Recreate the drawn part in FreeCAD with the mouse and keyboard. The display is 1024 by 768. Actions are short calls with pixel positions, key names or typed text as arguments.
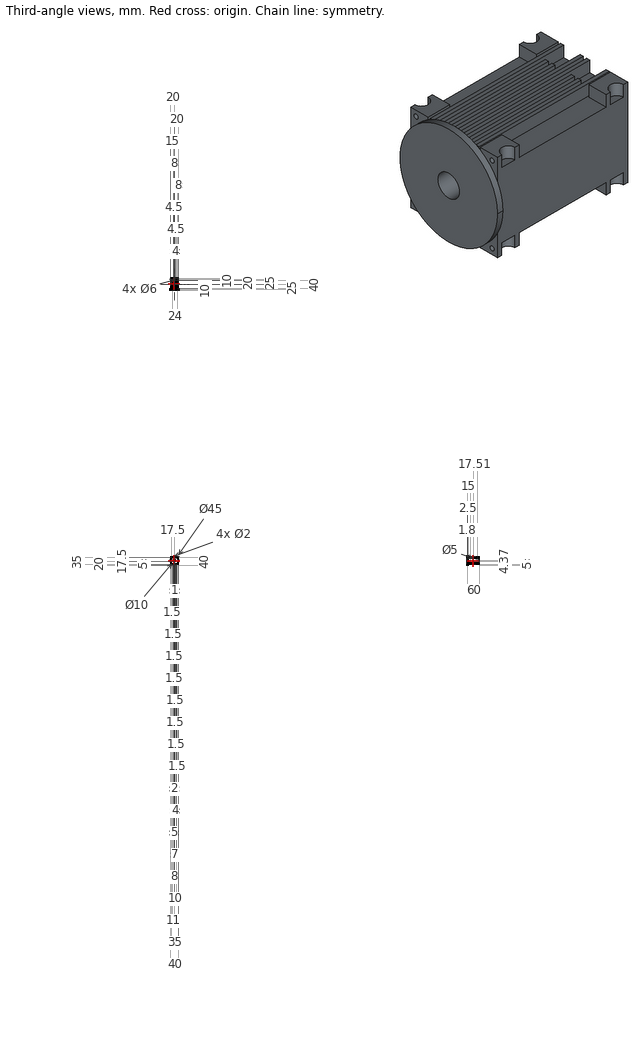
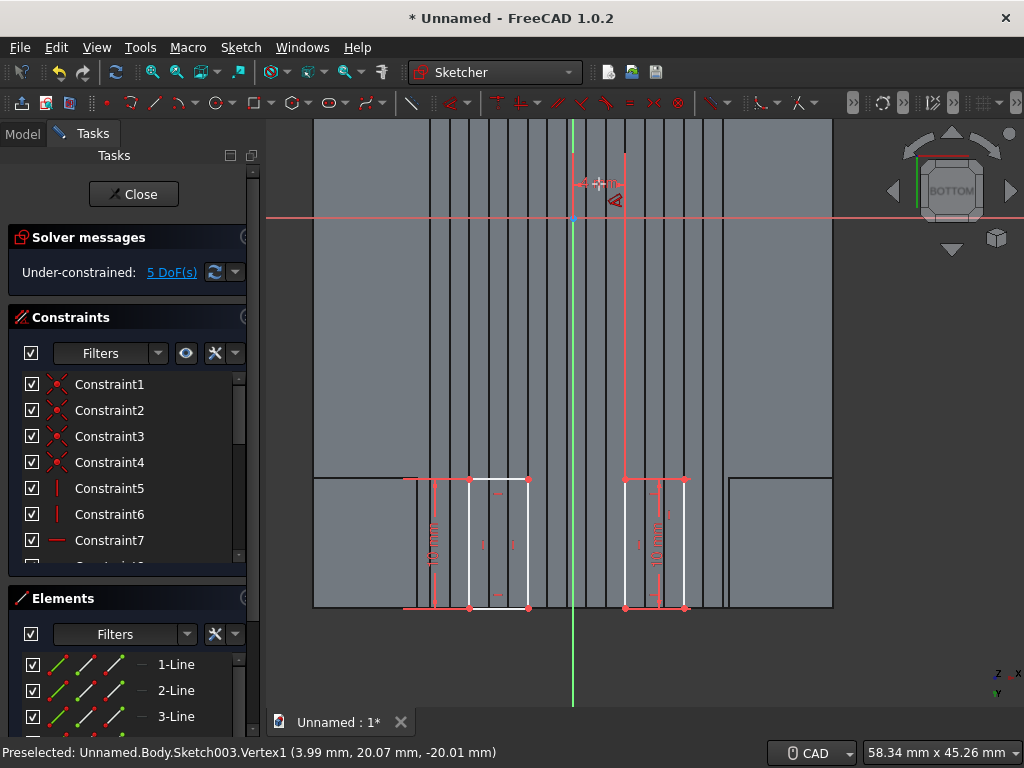
click(469, 479)
click(521, 184)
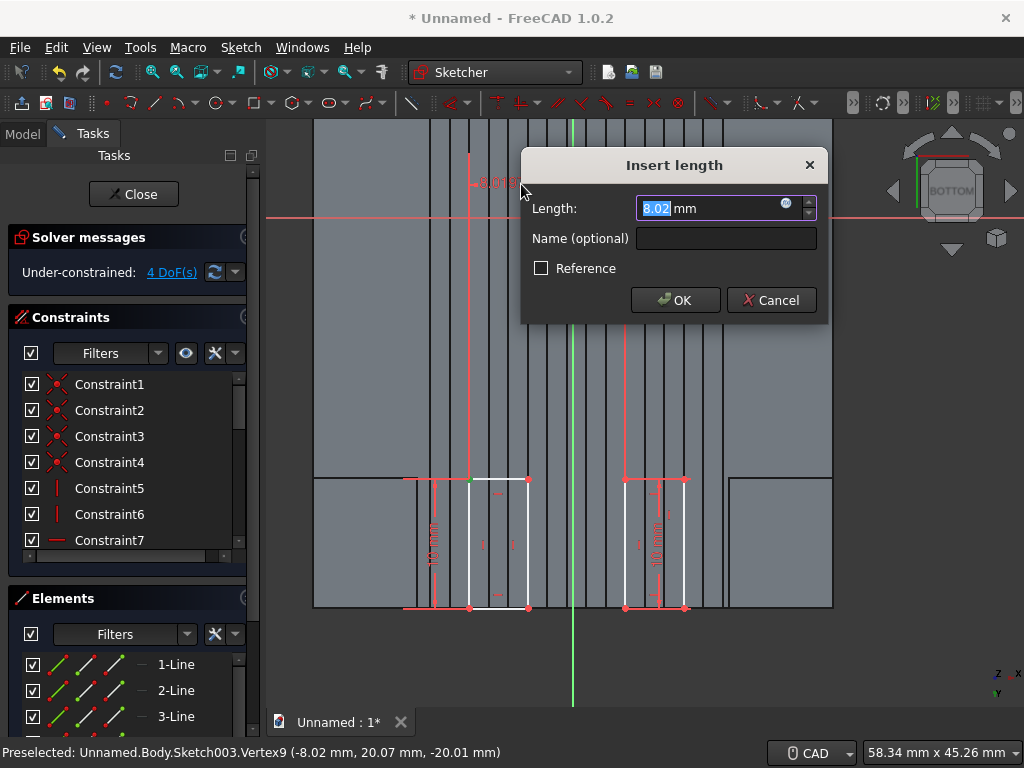
text(8)
key(Return)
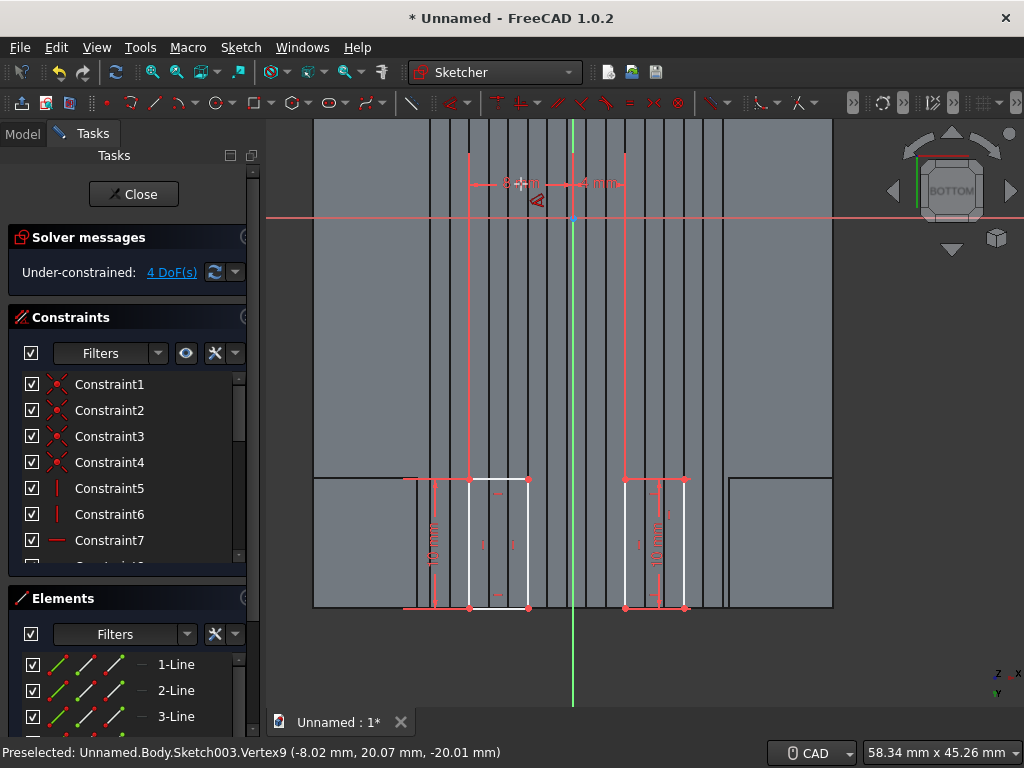
click(643, 609)
click(655, 643)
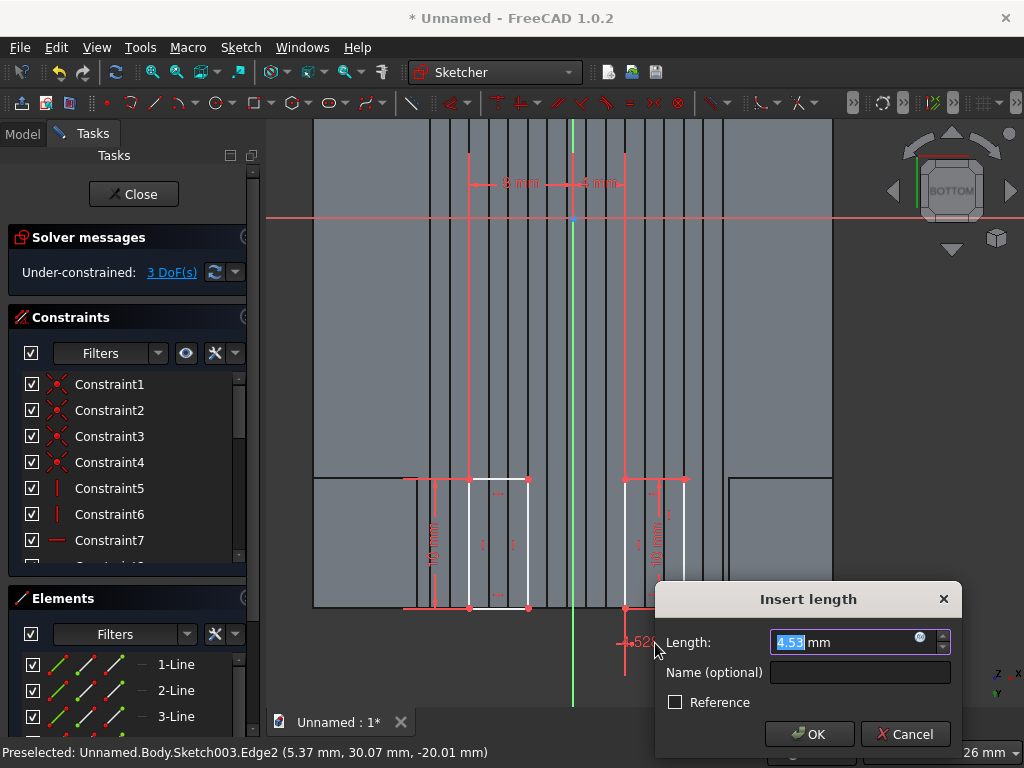
text(4.5)
key(Return)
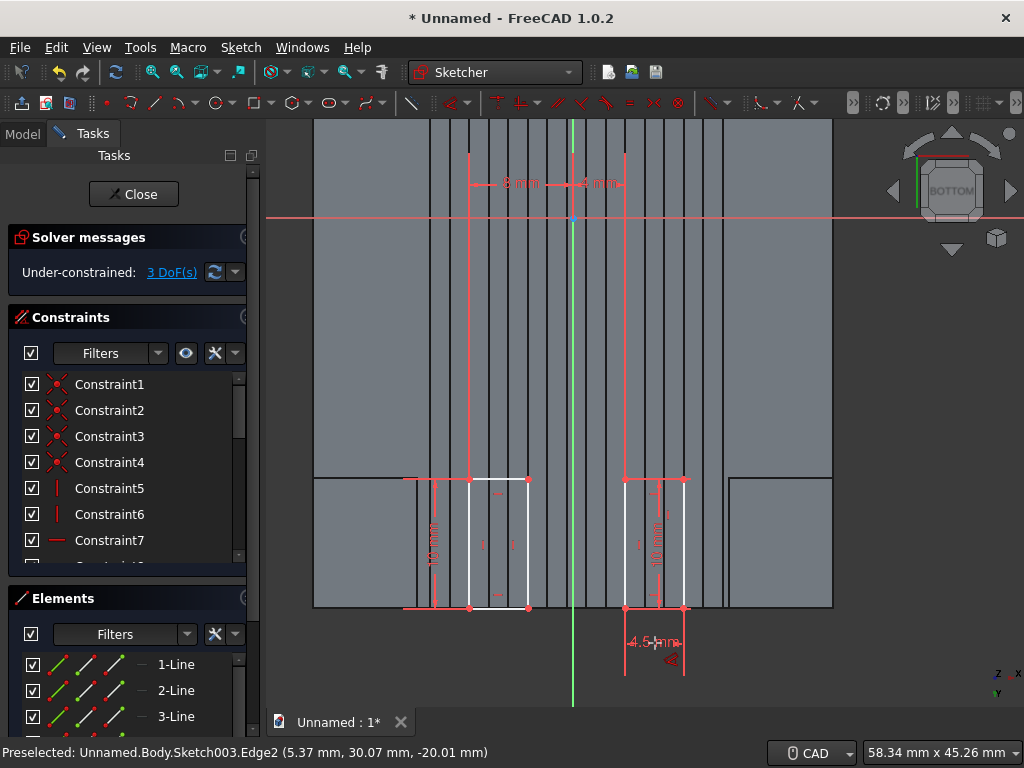
click(487, 609)
click(499, 643)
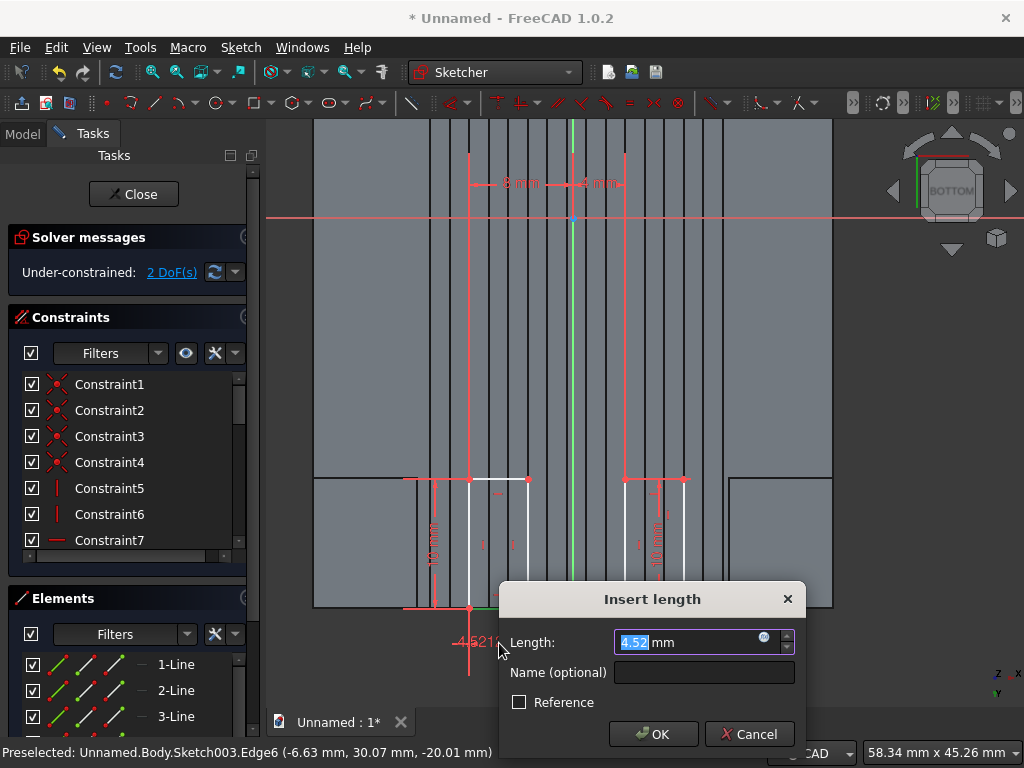
text(4.5)
key(Return)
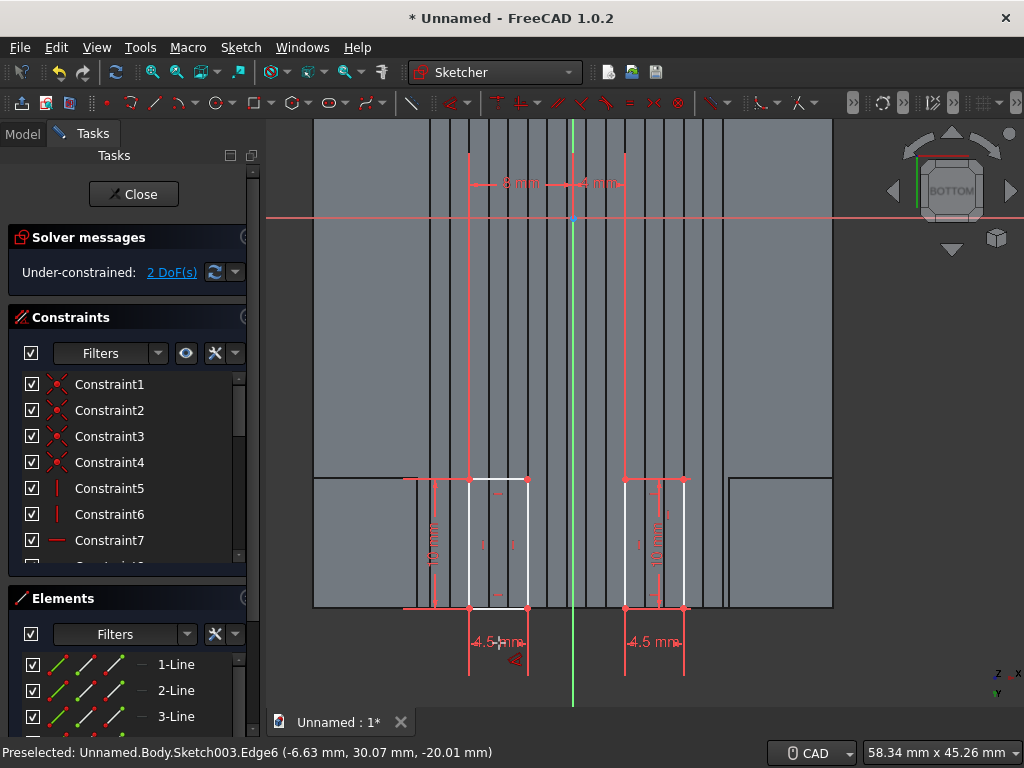
click(625, 479)
click(659, 349)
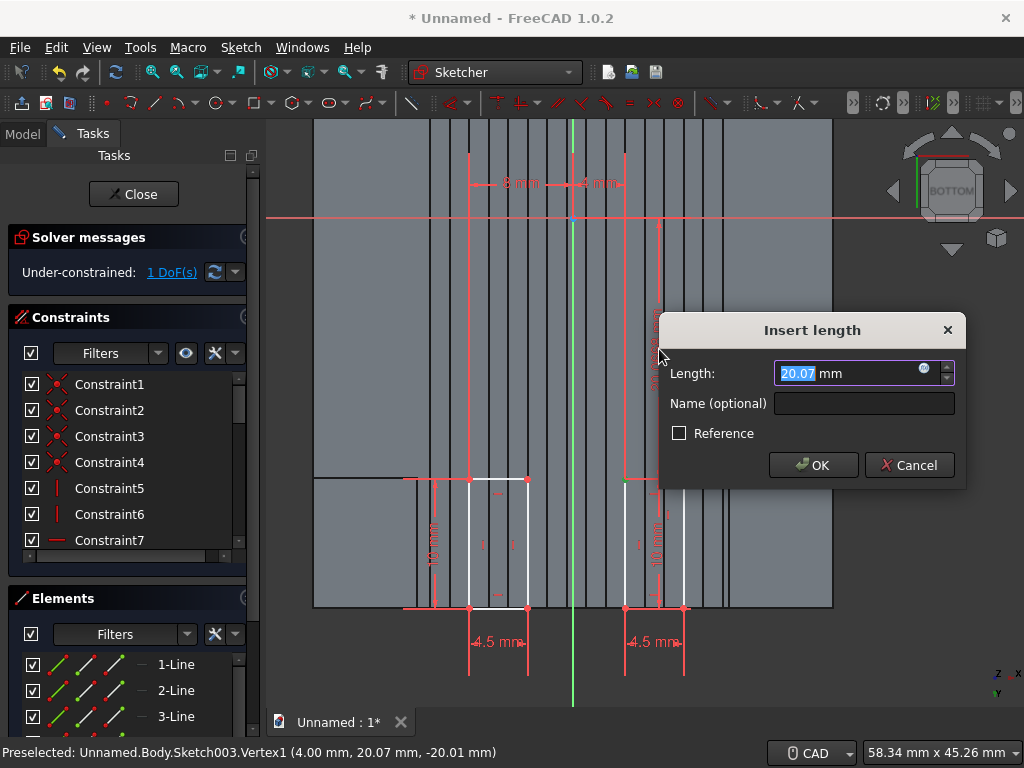
text(20)
key(Return)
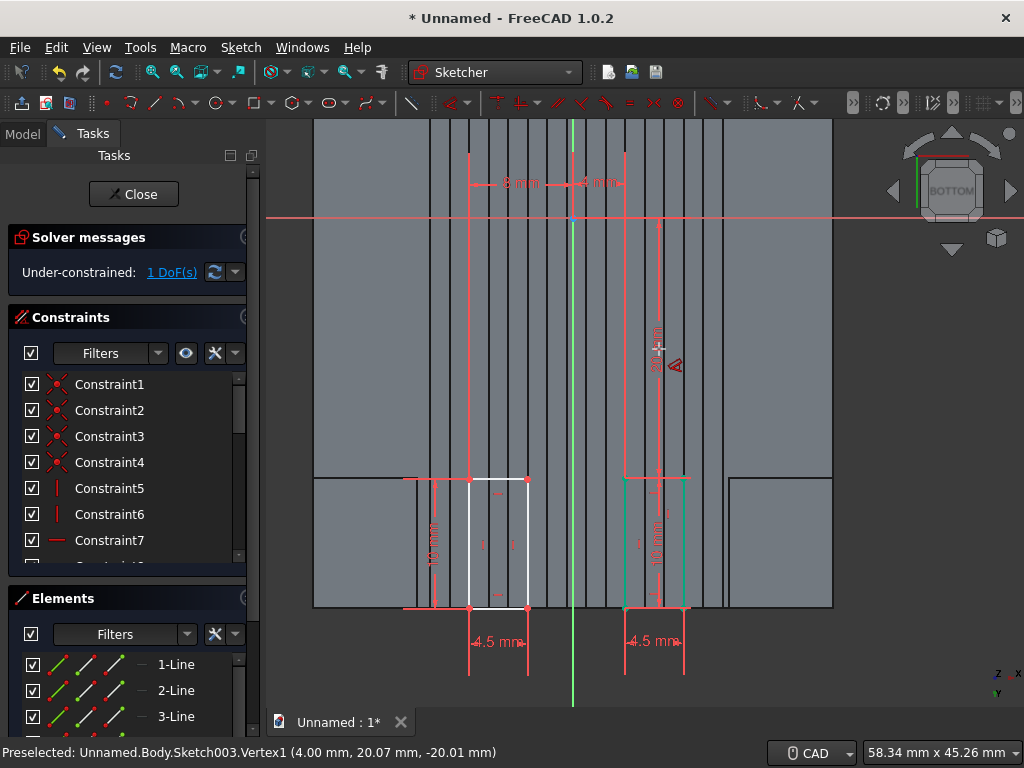
click(469, 479)
click(435, 349)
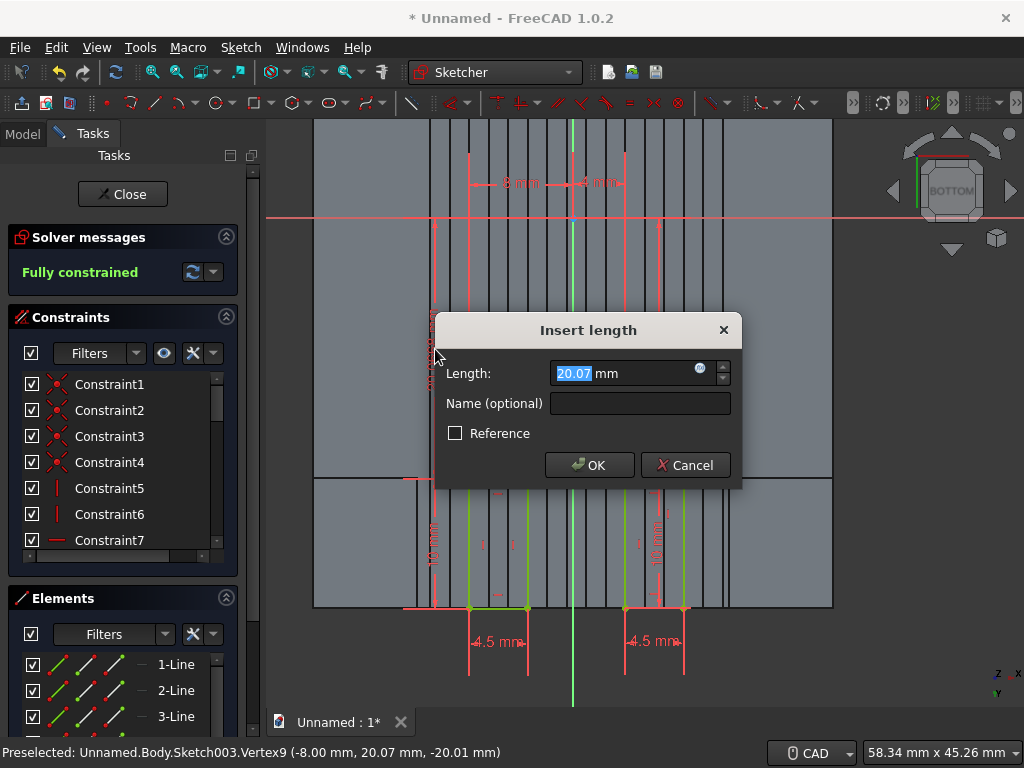
text(20)
key(Return)
key(Escape)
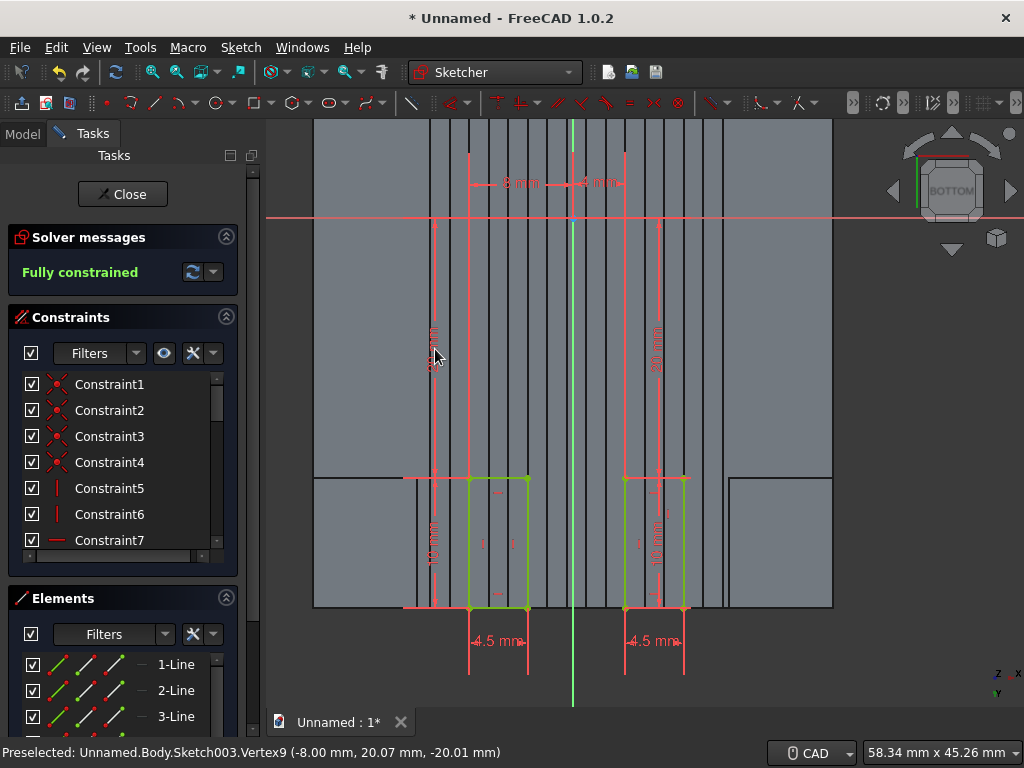
click(123, 194)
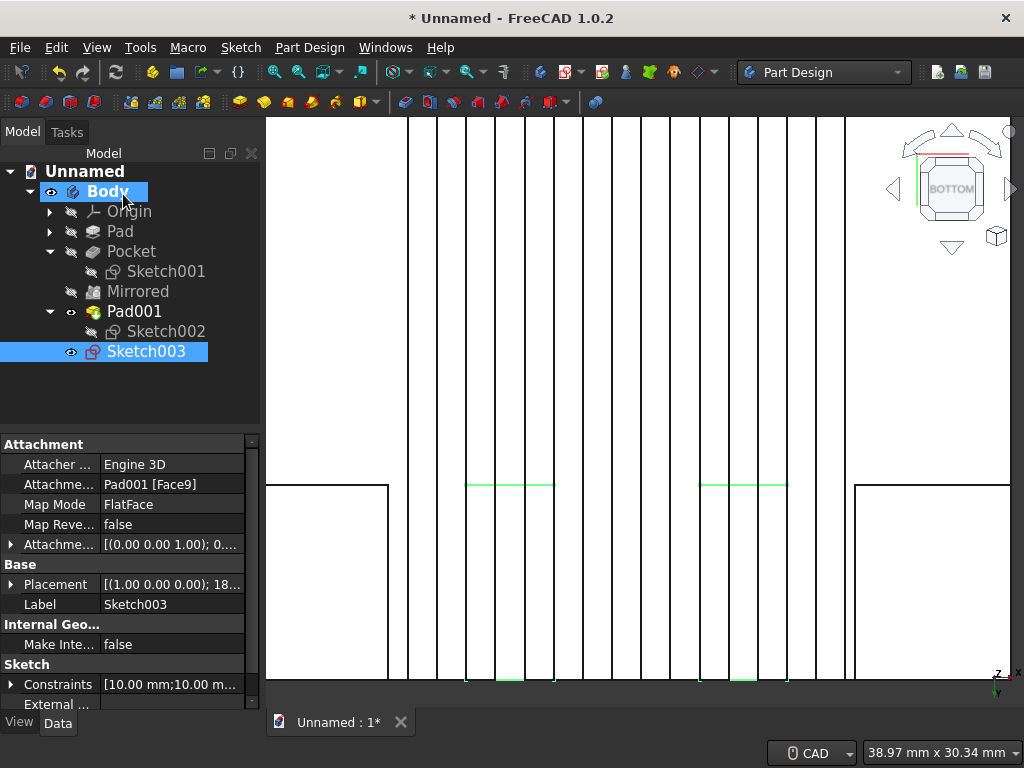
click(406, 102)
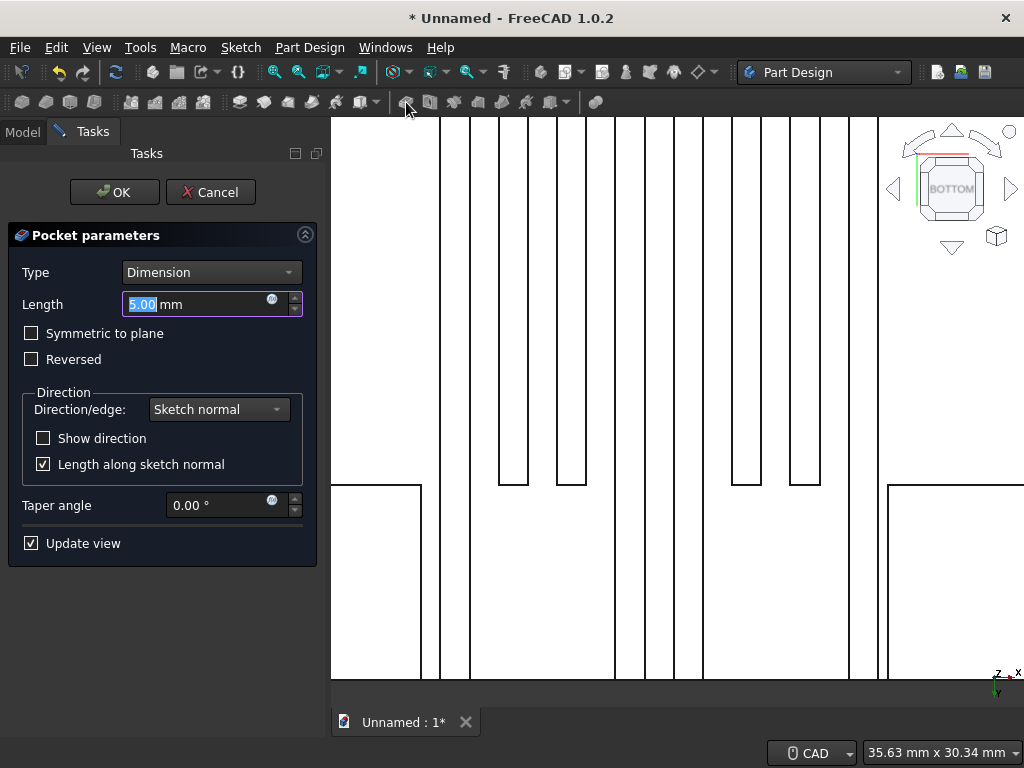
text(5)
key(Tab)